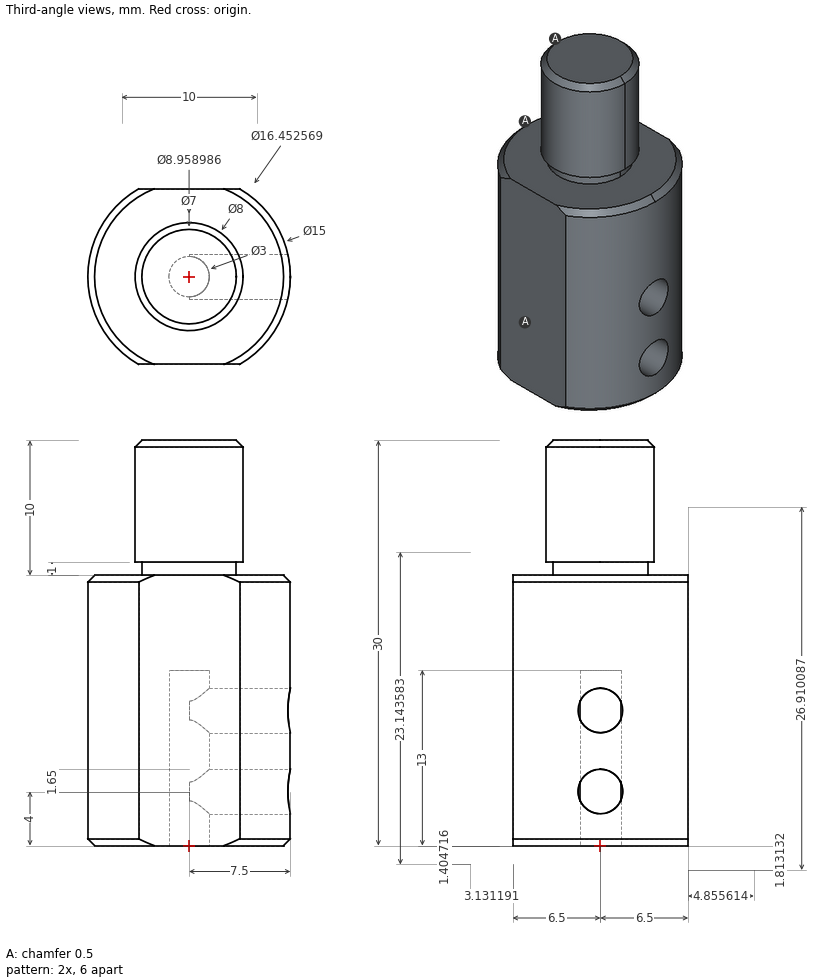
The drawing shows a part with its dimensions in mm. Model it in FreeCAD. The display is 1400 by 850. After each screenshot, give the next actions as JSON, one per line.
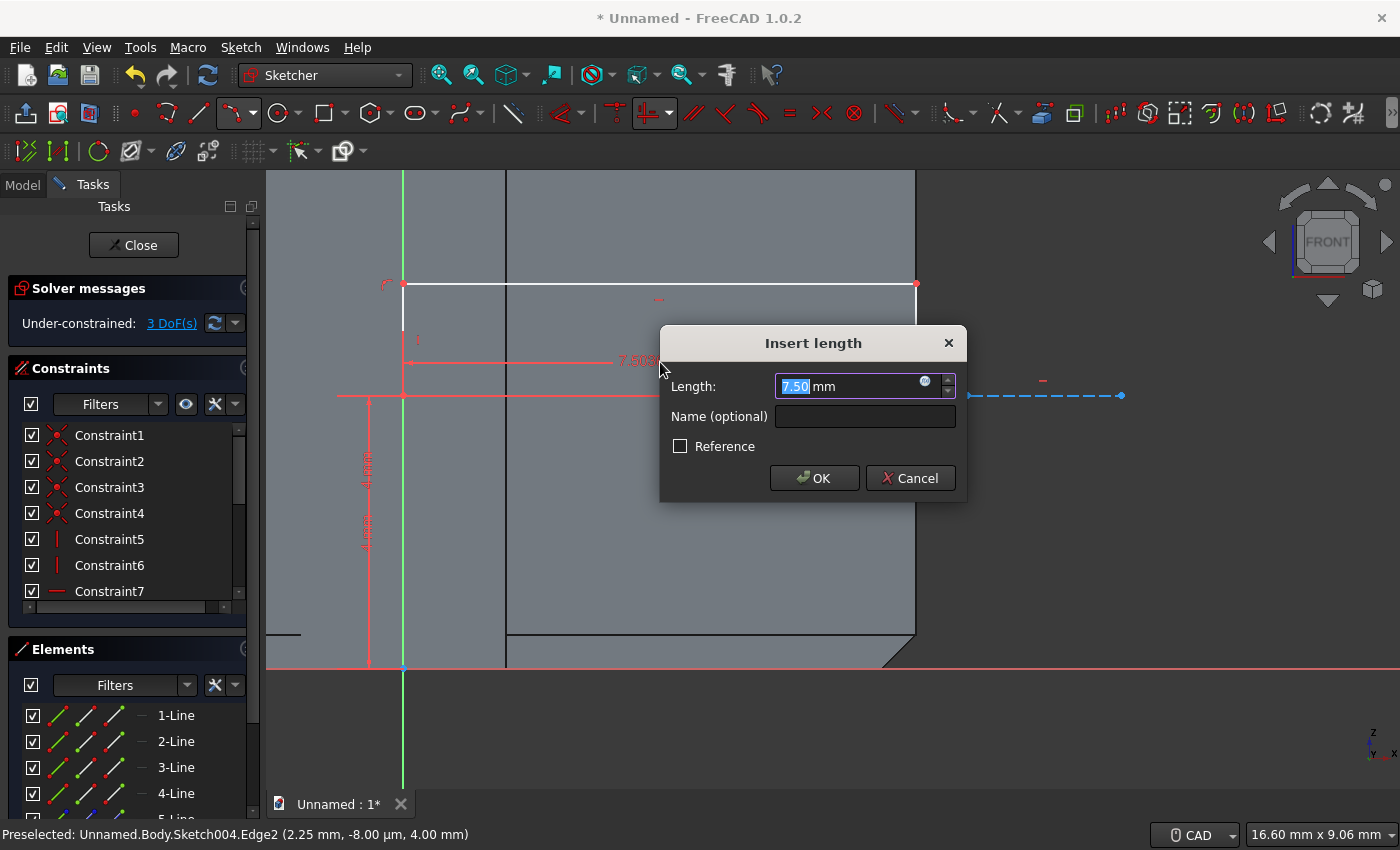
{"action": "type", "text": "7.5"}
{"action": "key", "text": "Return"}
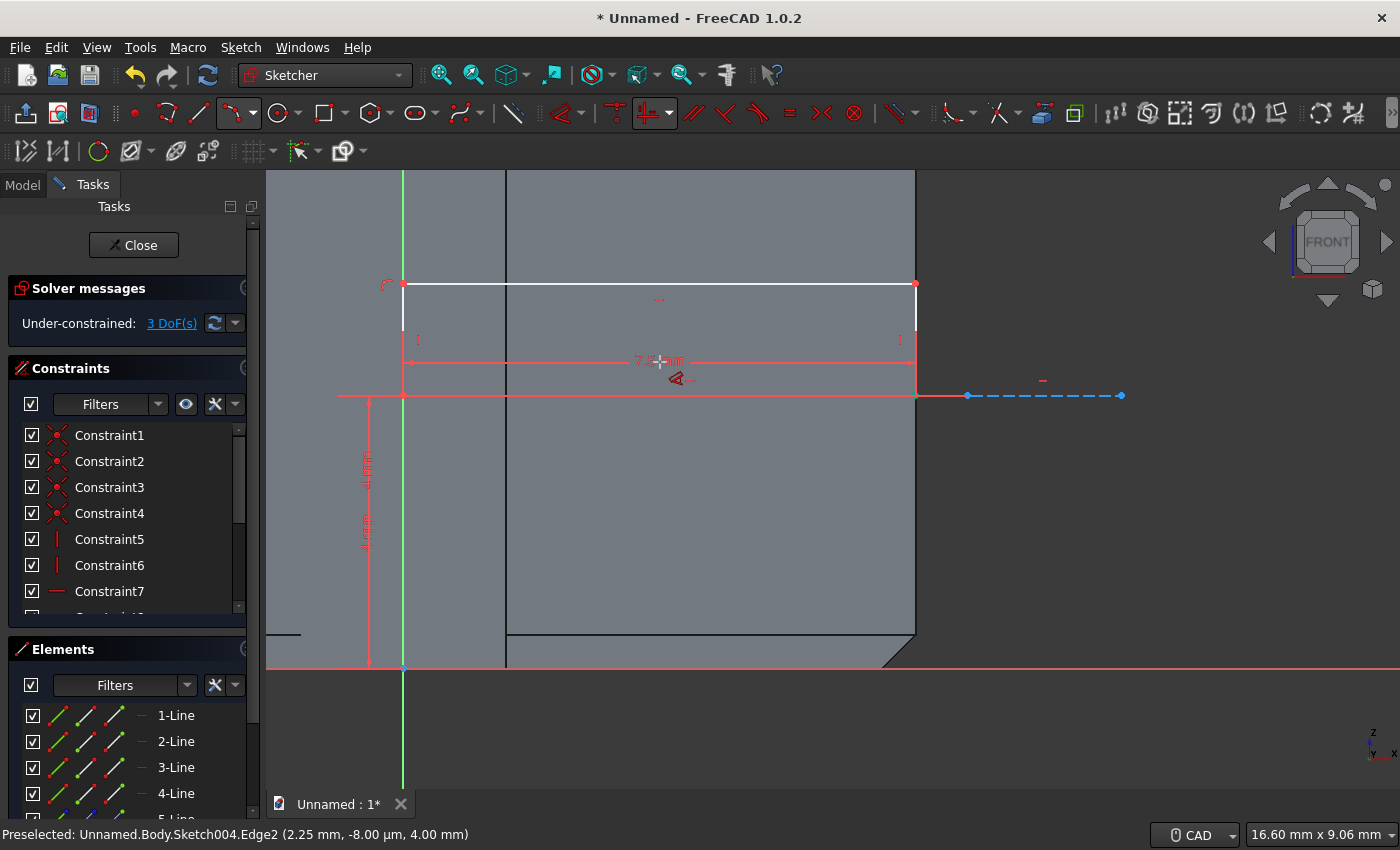
{"action": "left_click", "coordinate": [403, 317]}
{"action": "left_click", "coordinate": [369, 340]}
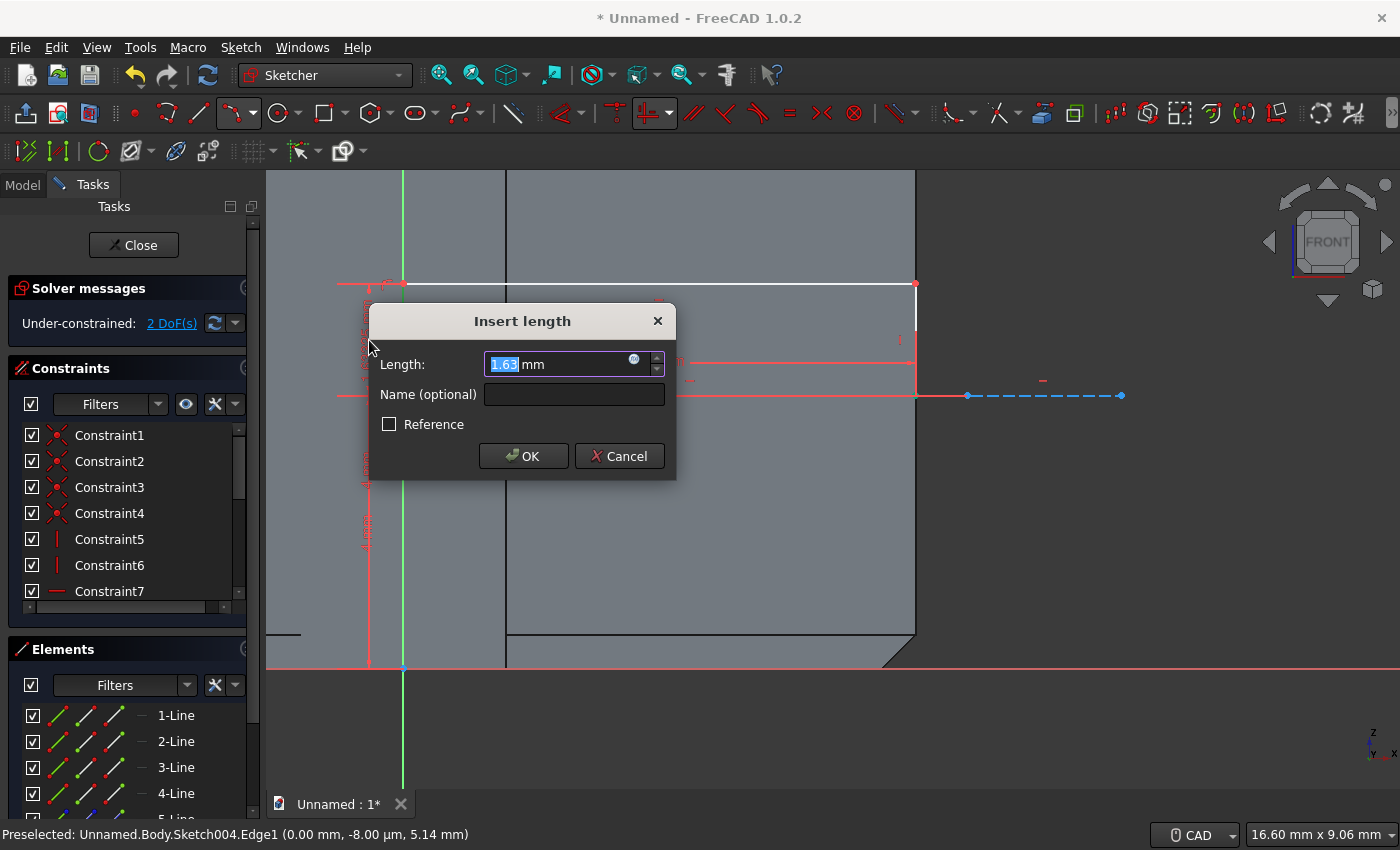
{"action": "type", "text": "1.65"}
{"action": "key", "text": "Return"}
{"action": "key", "text": "Escape"}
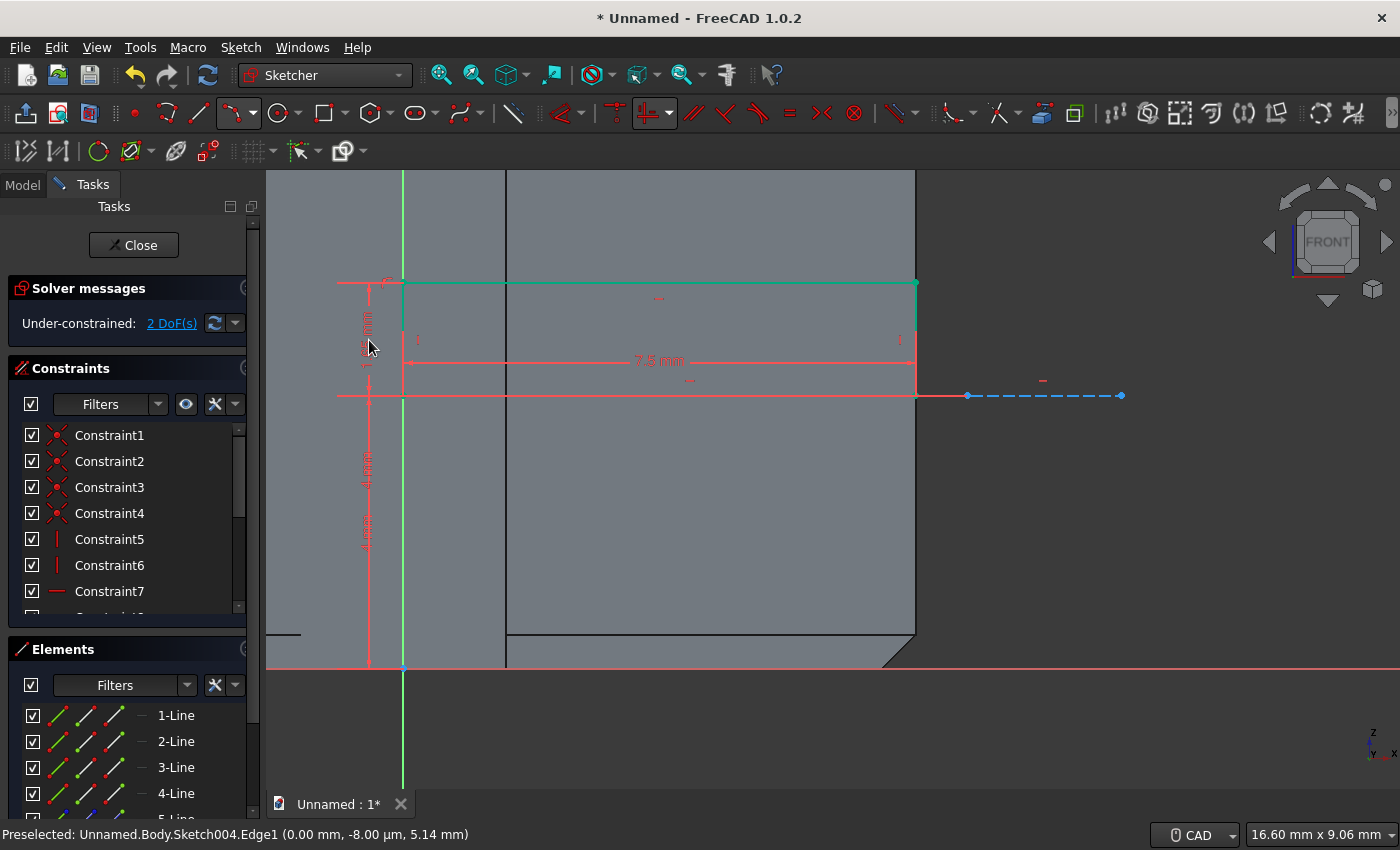
{"action": "left_click", "coordinate": [134, 245]}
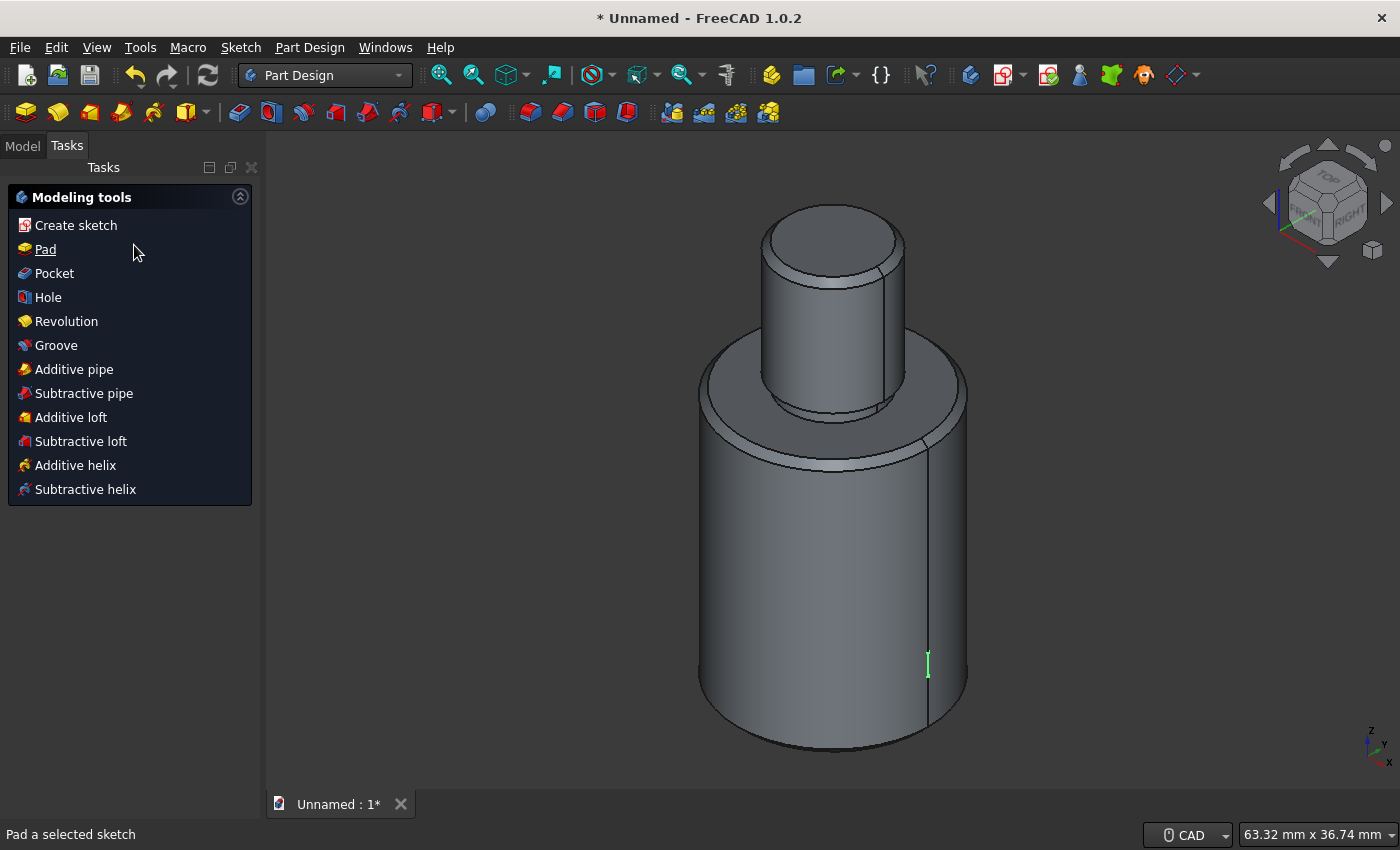
{"action": "left_click", "coordinate": [304, 112]}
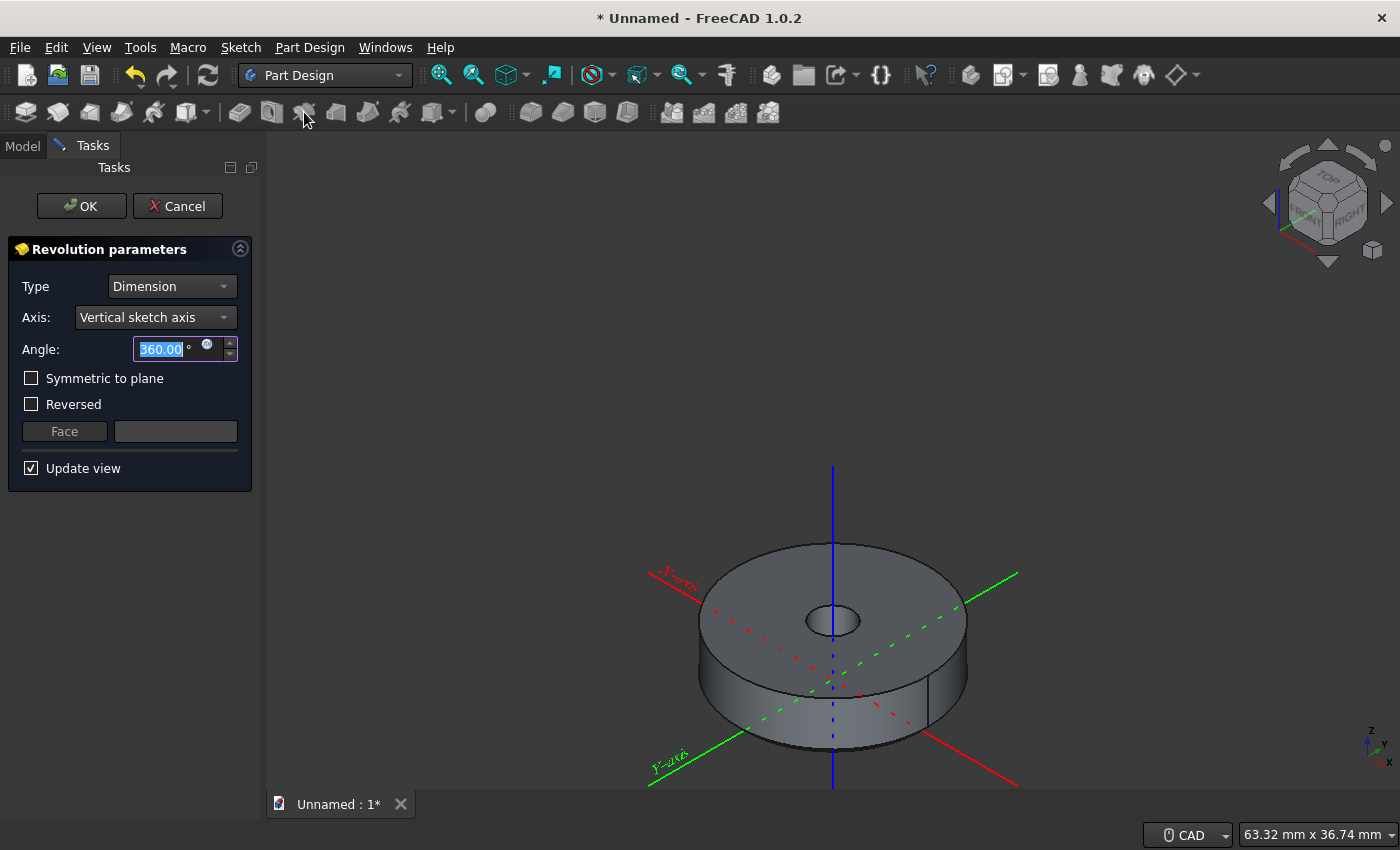
{"action": "left_click", "coordinate": [156, 318]}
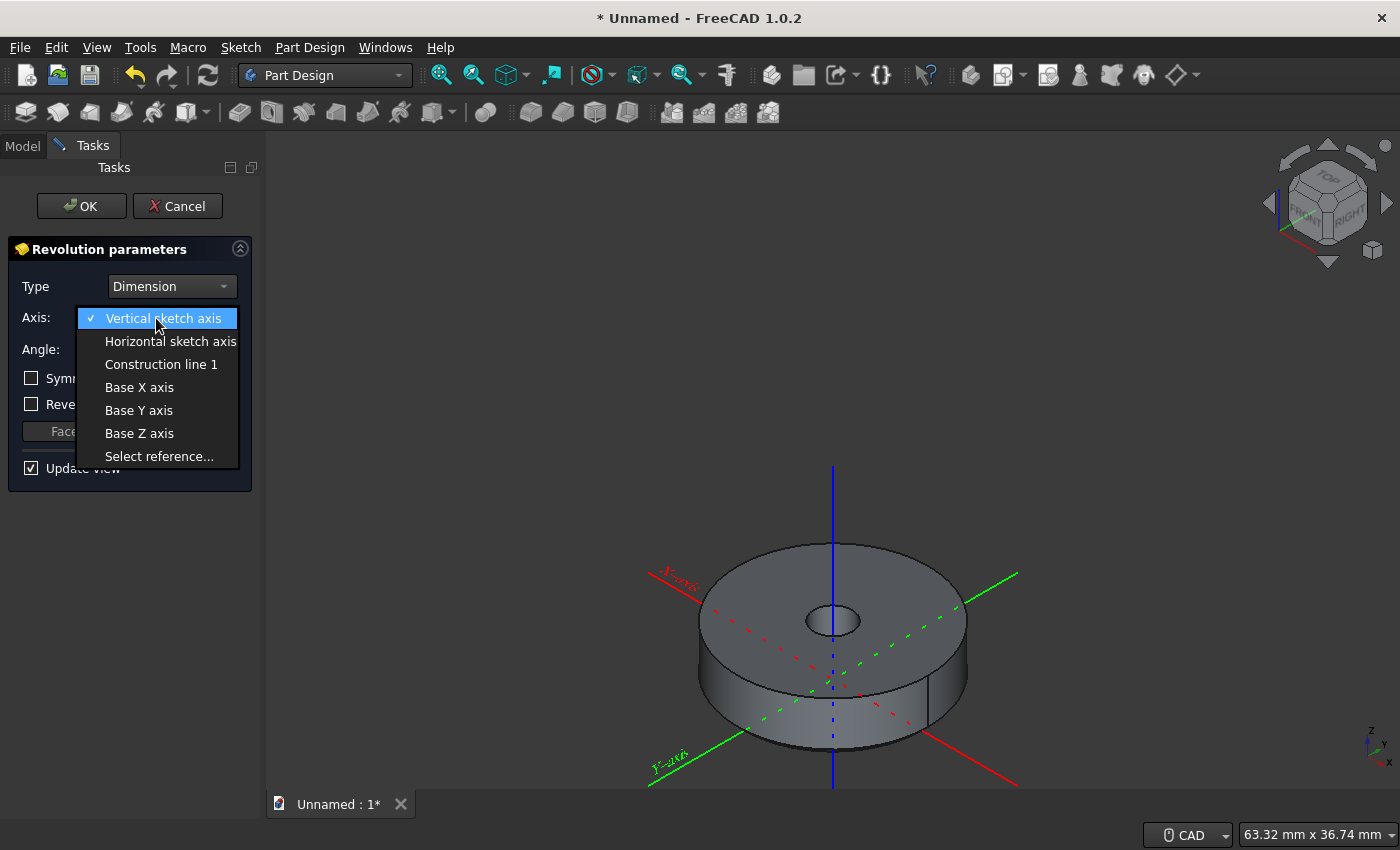
{"action": "left_click", "coordinate": [156, 364]}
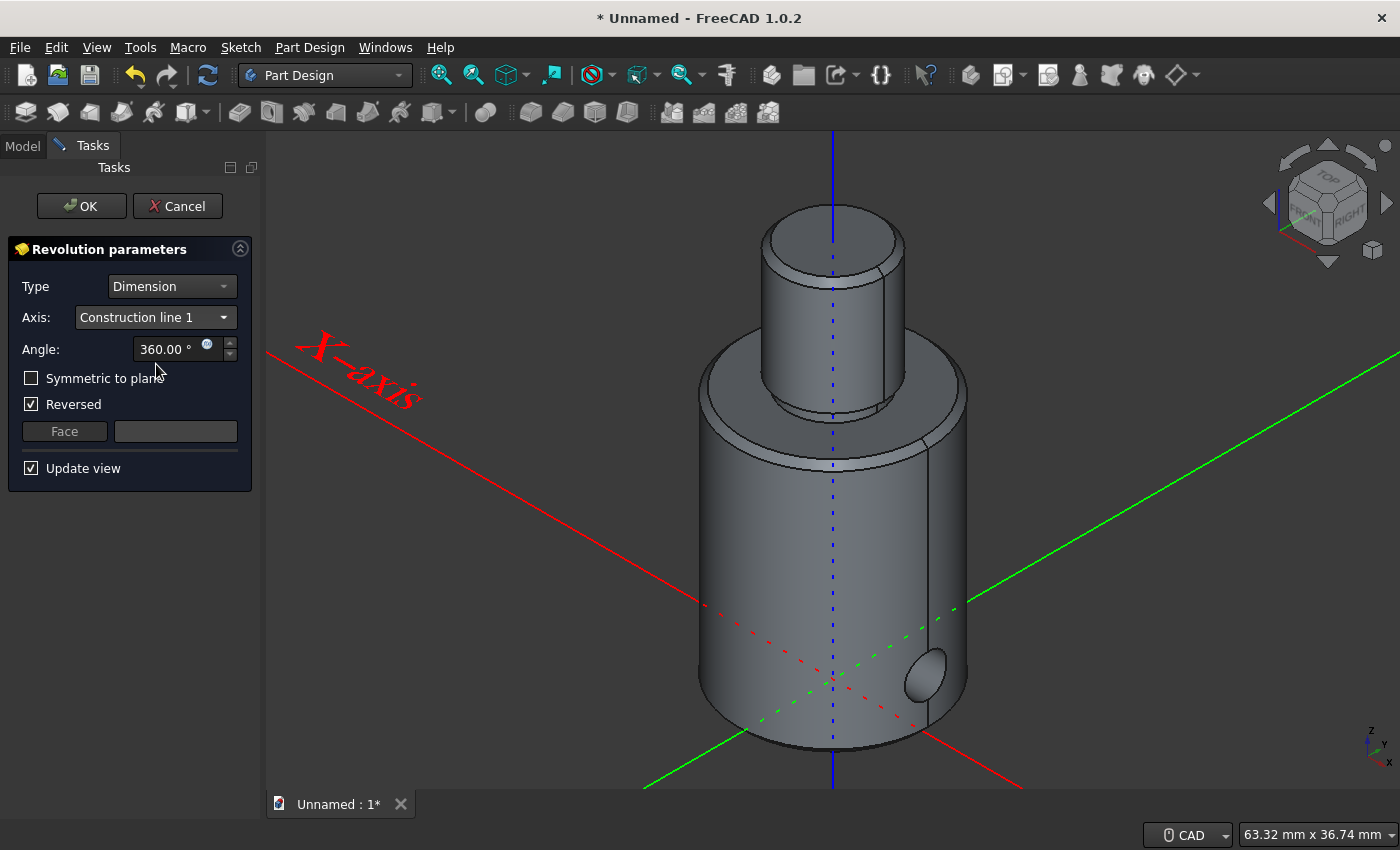
{"action": "left_click", "coordinate": [82, 206]}